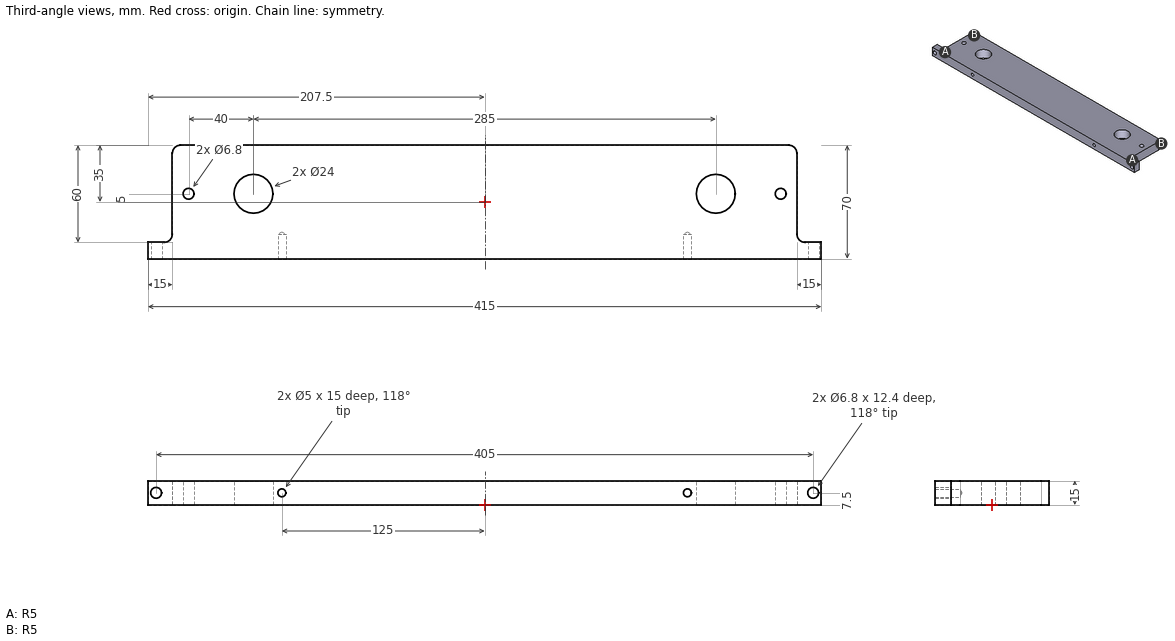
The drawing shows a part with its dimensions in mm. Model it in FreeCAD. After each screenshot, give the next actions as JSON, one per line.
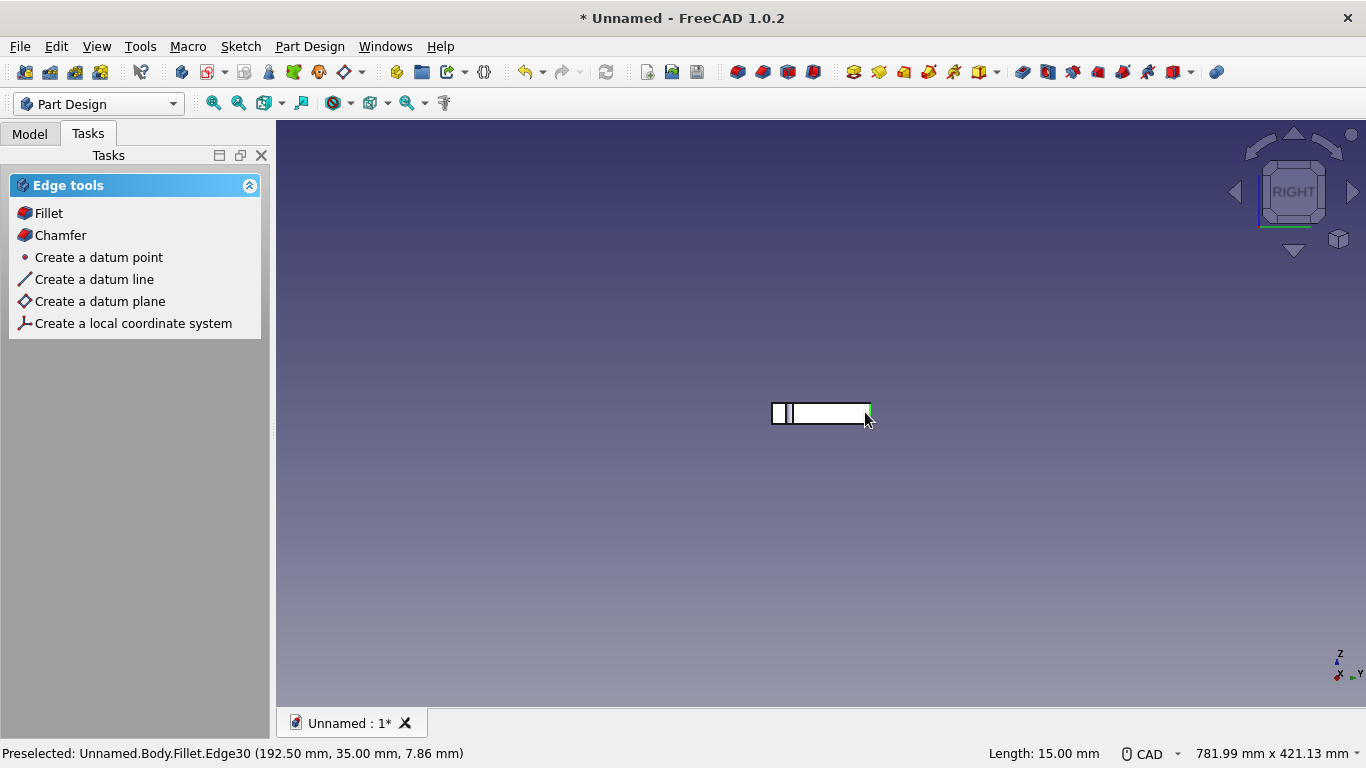
{"action": "scroll", "coordinate": [870, 412], "scroll_direction": "up", "scroll_amount": 4}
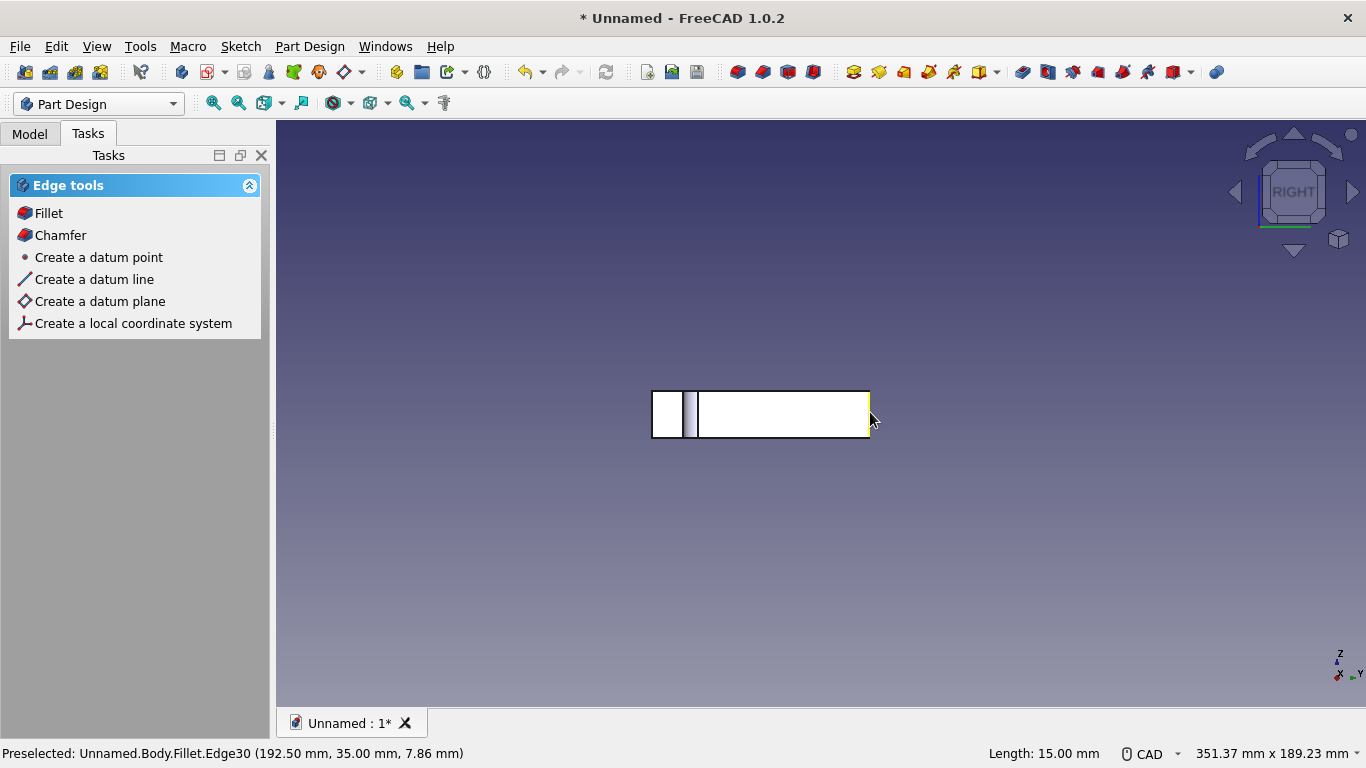
{"action": "left_click", "coordinate": [214, 104]}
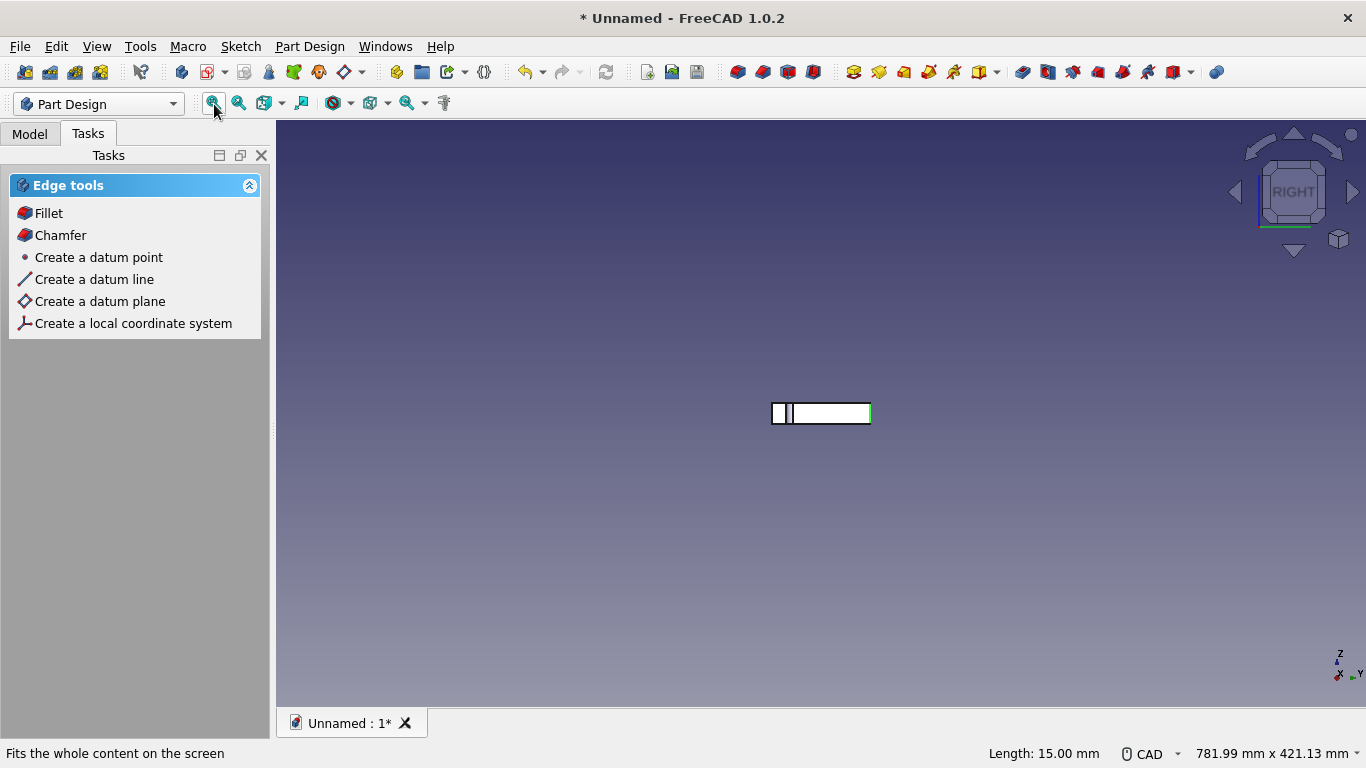
{"action": "key", "text": "5"}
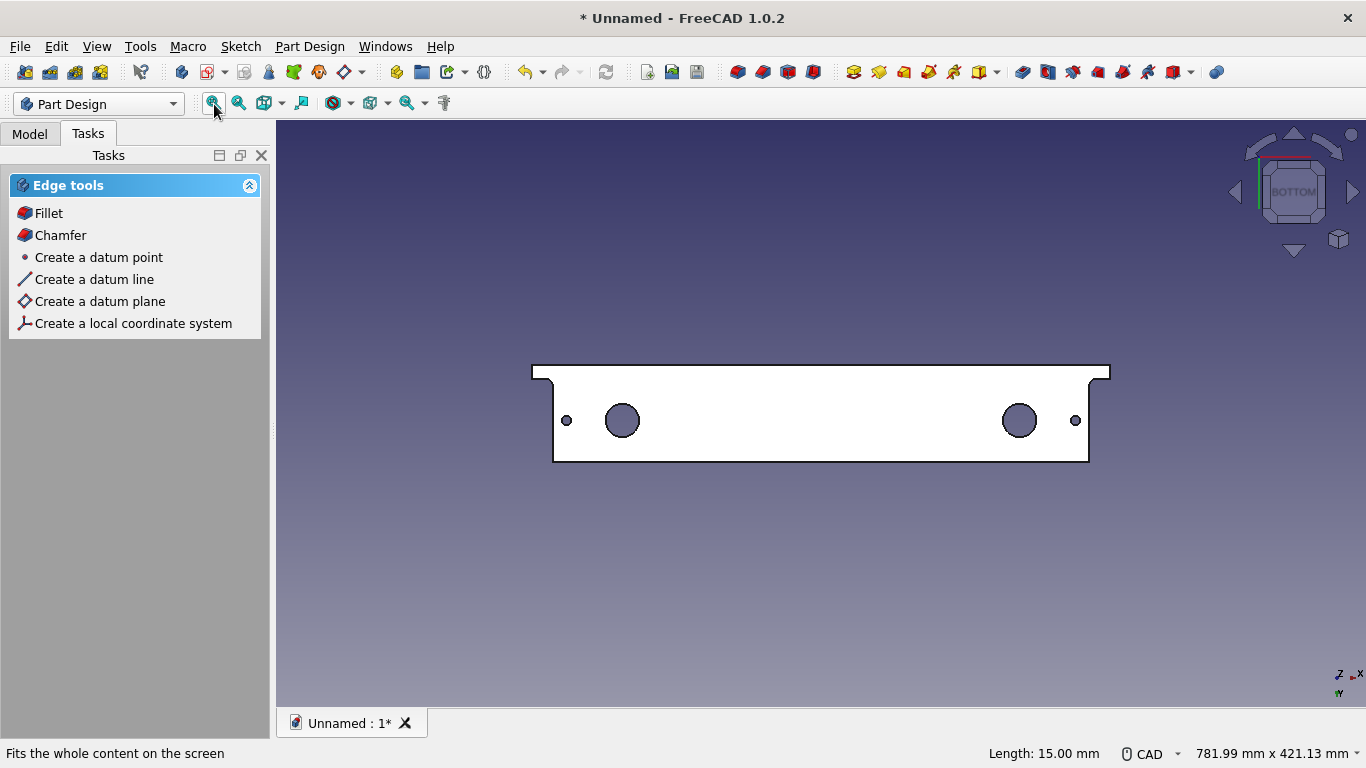
{"action": "scroll", "coordinate": [553, 461], "scroll_direction": "up", "scroll_amount": 4}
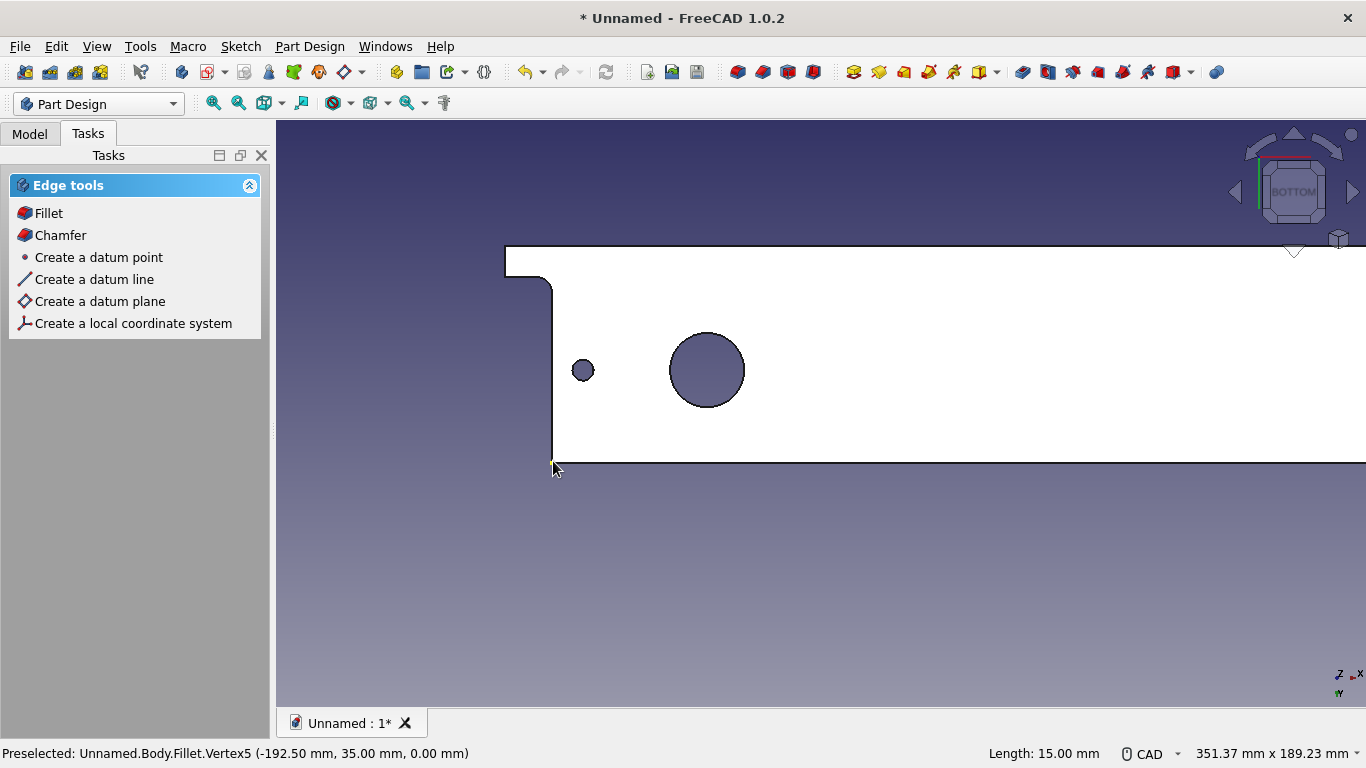
{"action": "key", "text": "v f"}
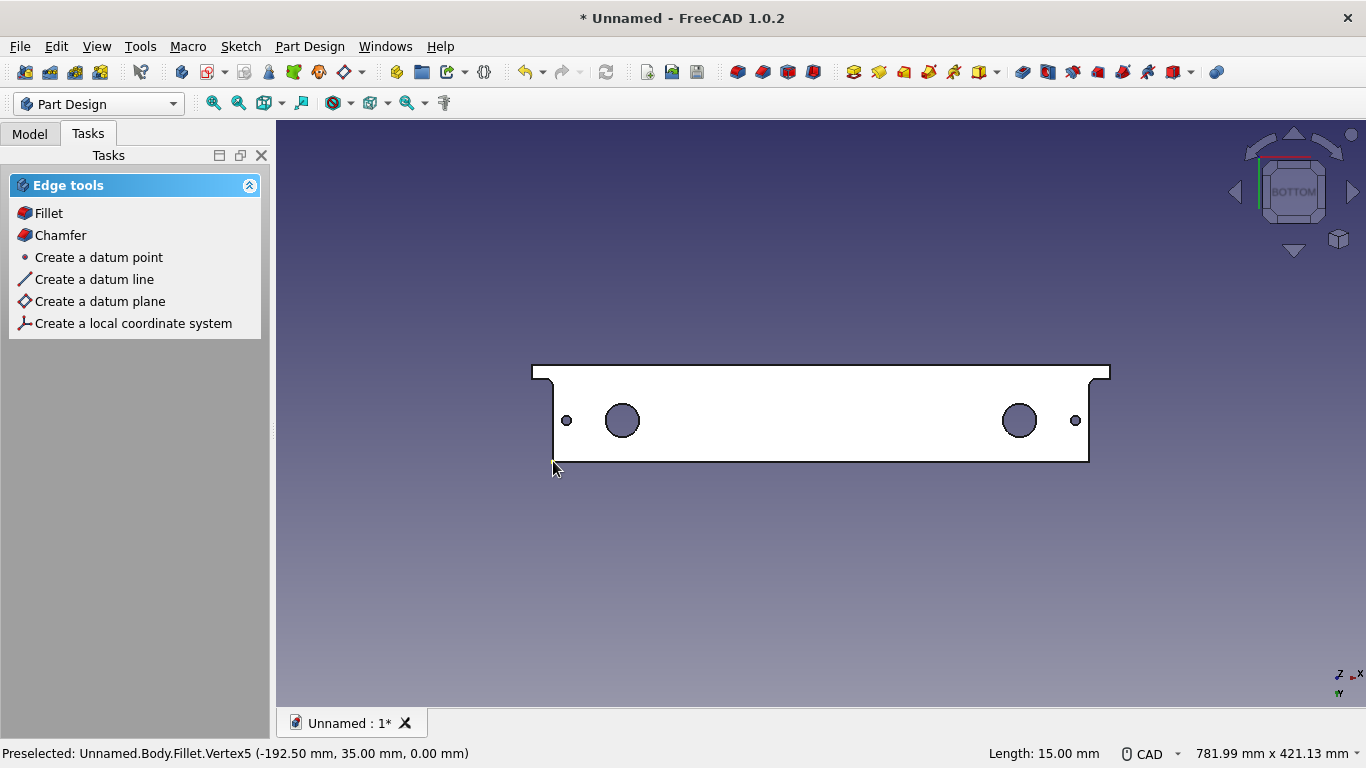
{"action": "key", "text": "4"}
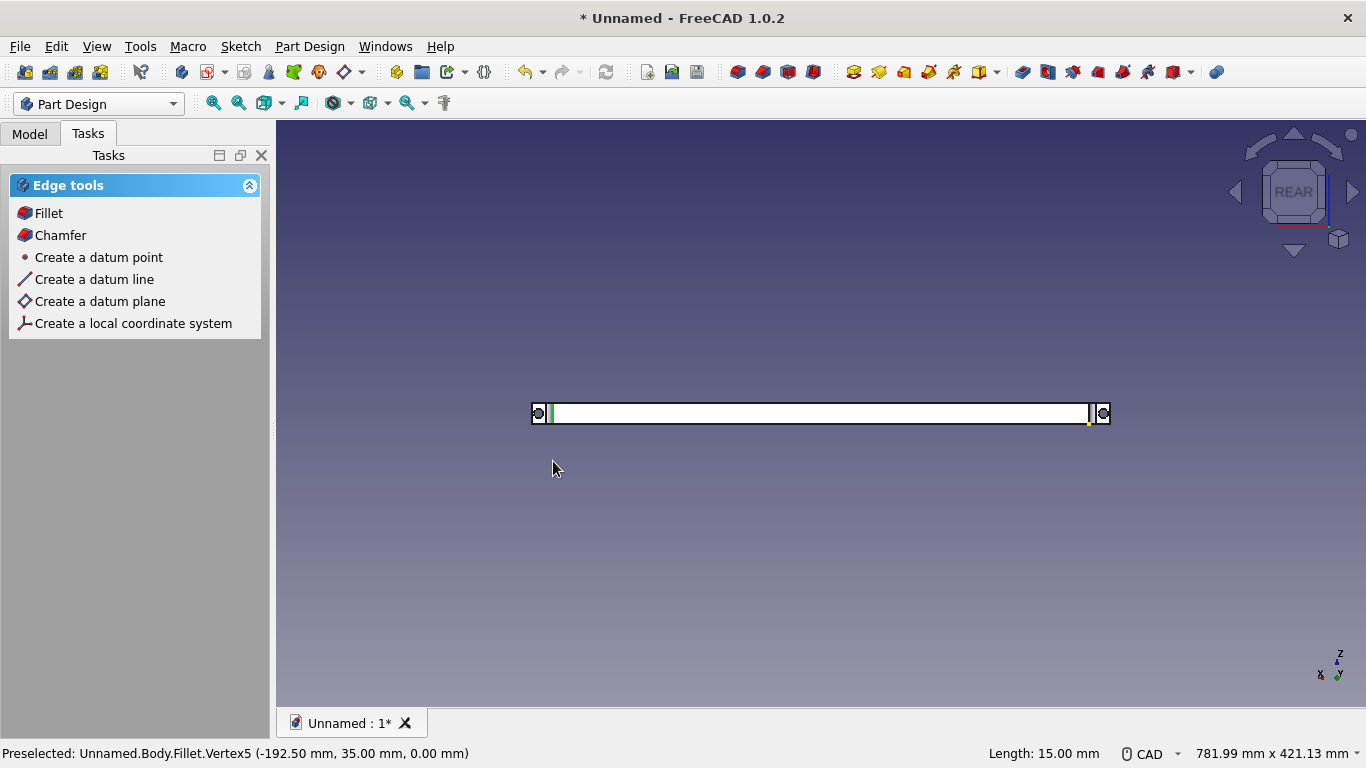
{"action": "left_click", "coordinate": [1089, 412], "text": "ctrl"}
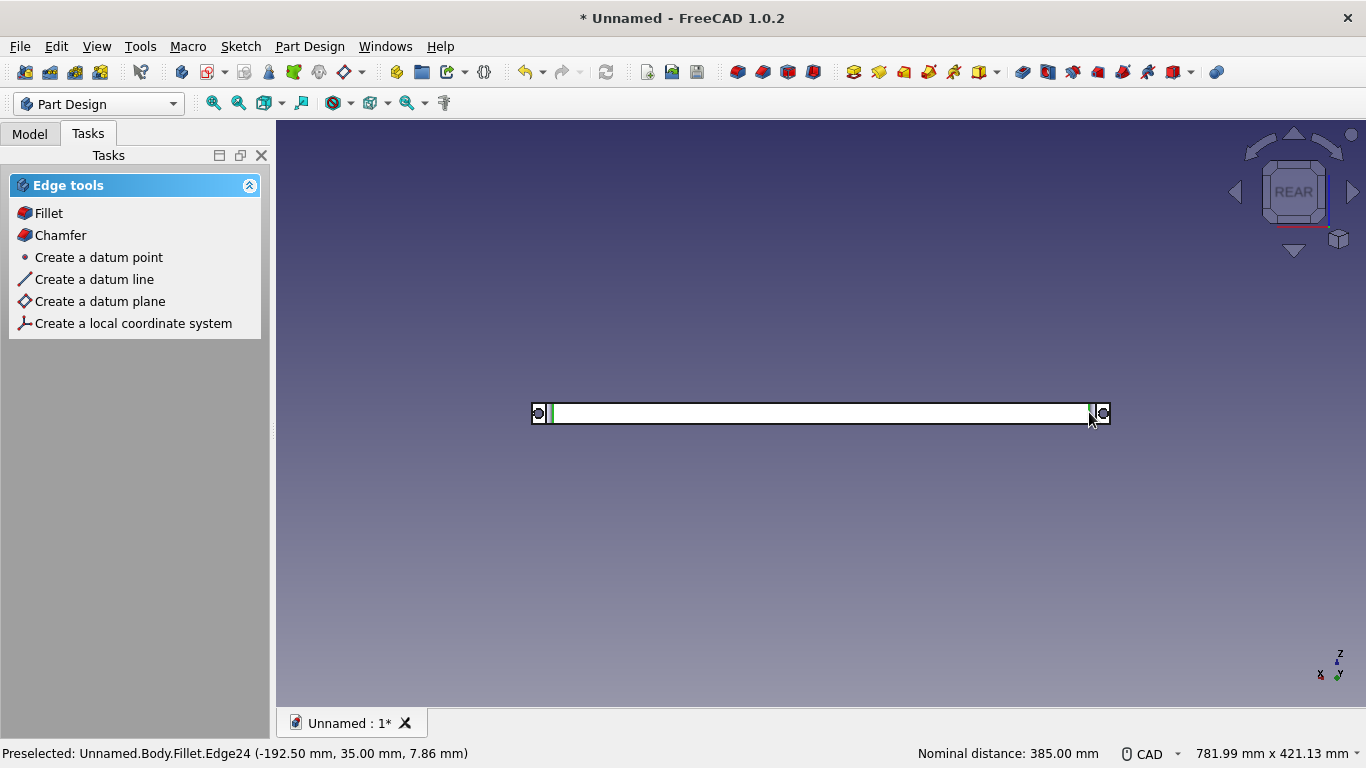
{"action": "left_click", "coordinate": [738, 72]}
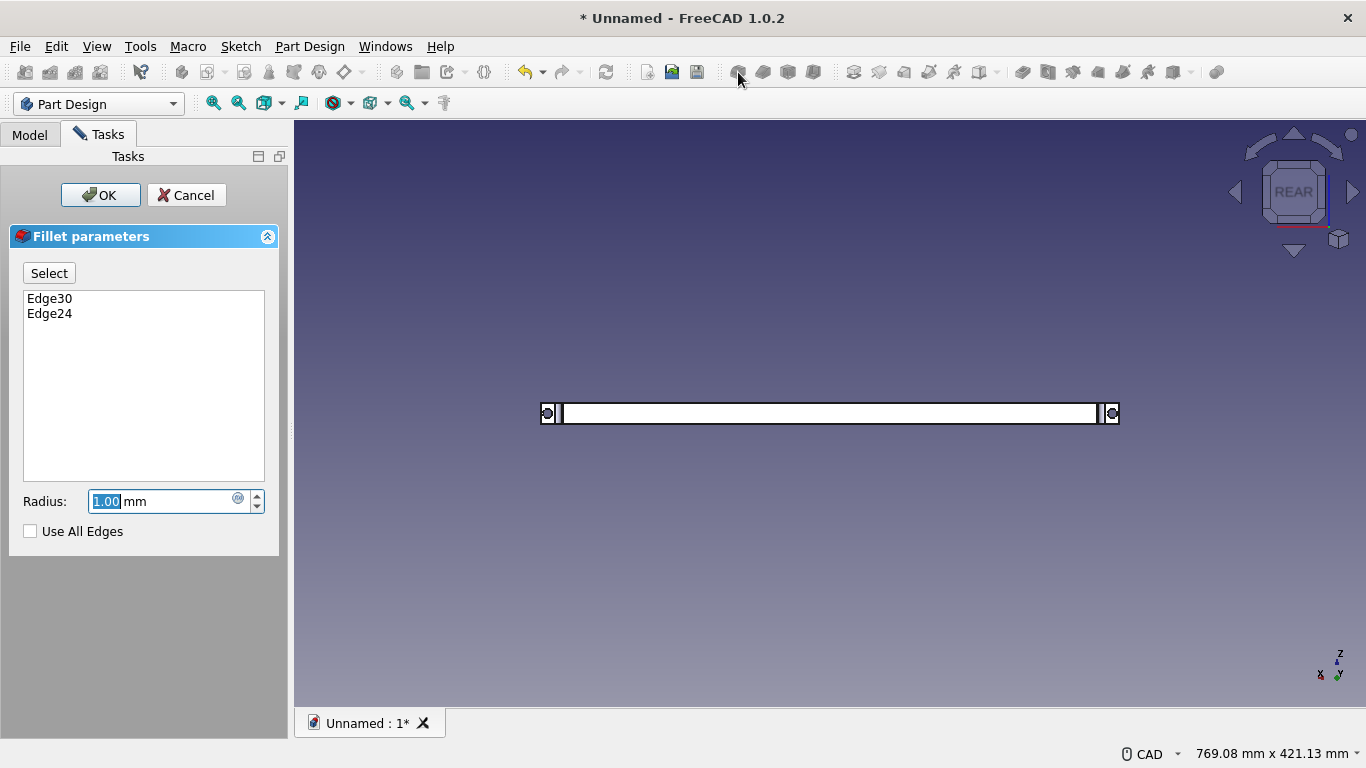
{"action": "type", "text": "5"}
{"action": "key", "text": "Tab"}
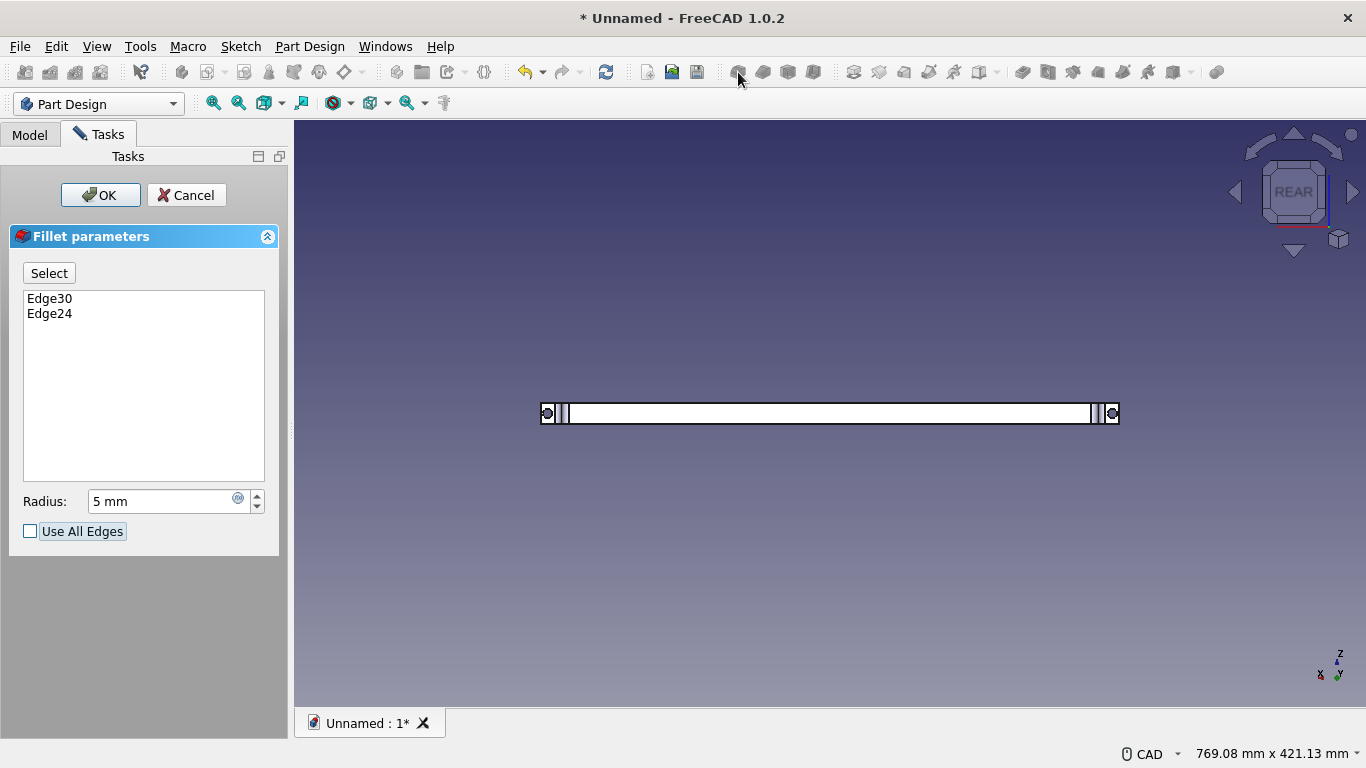
{"action": "left_click", "coordinate": [101, 195]}